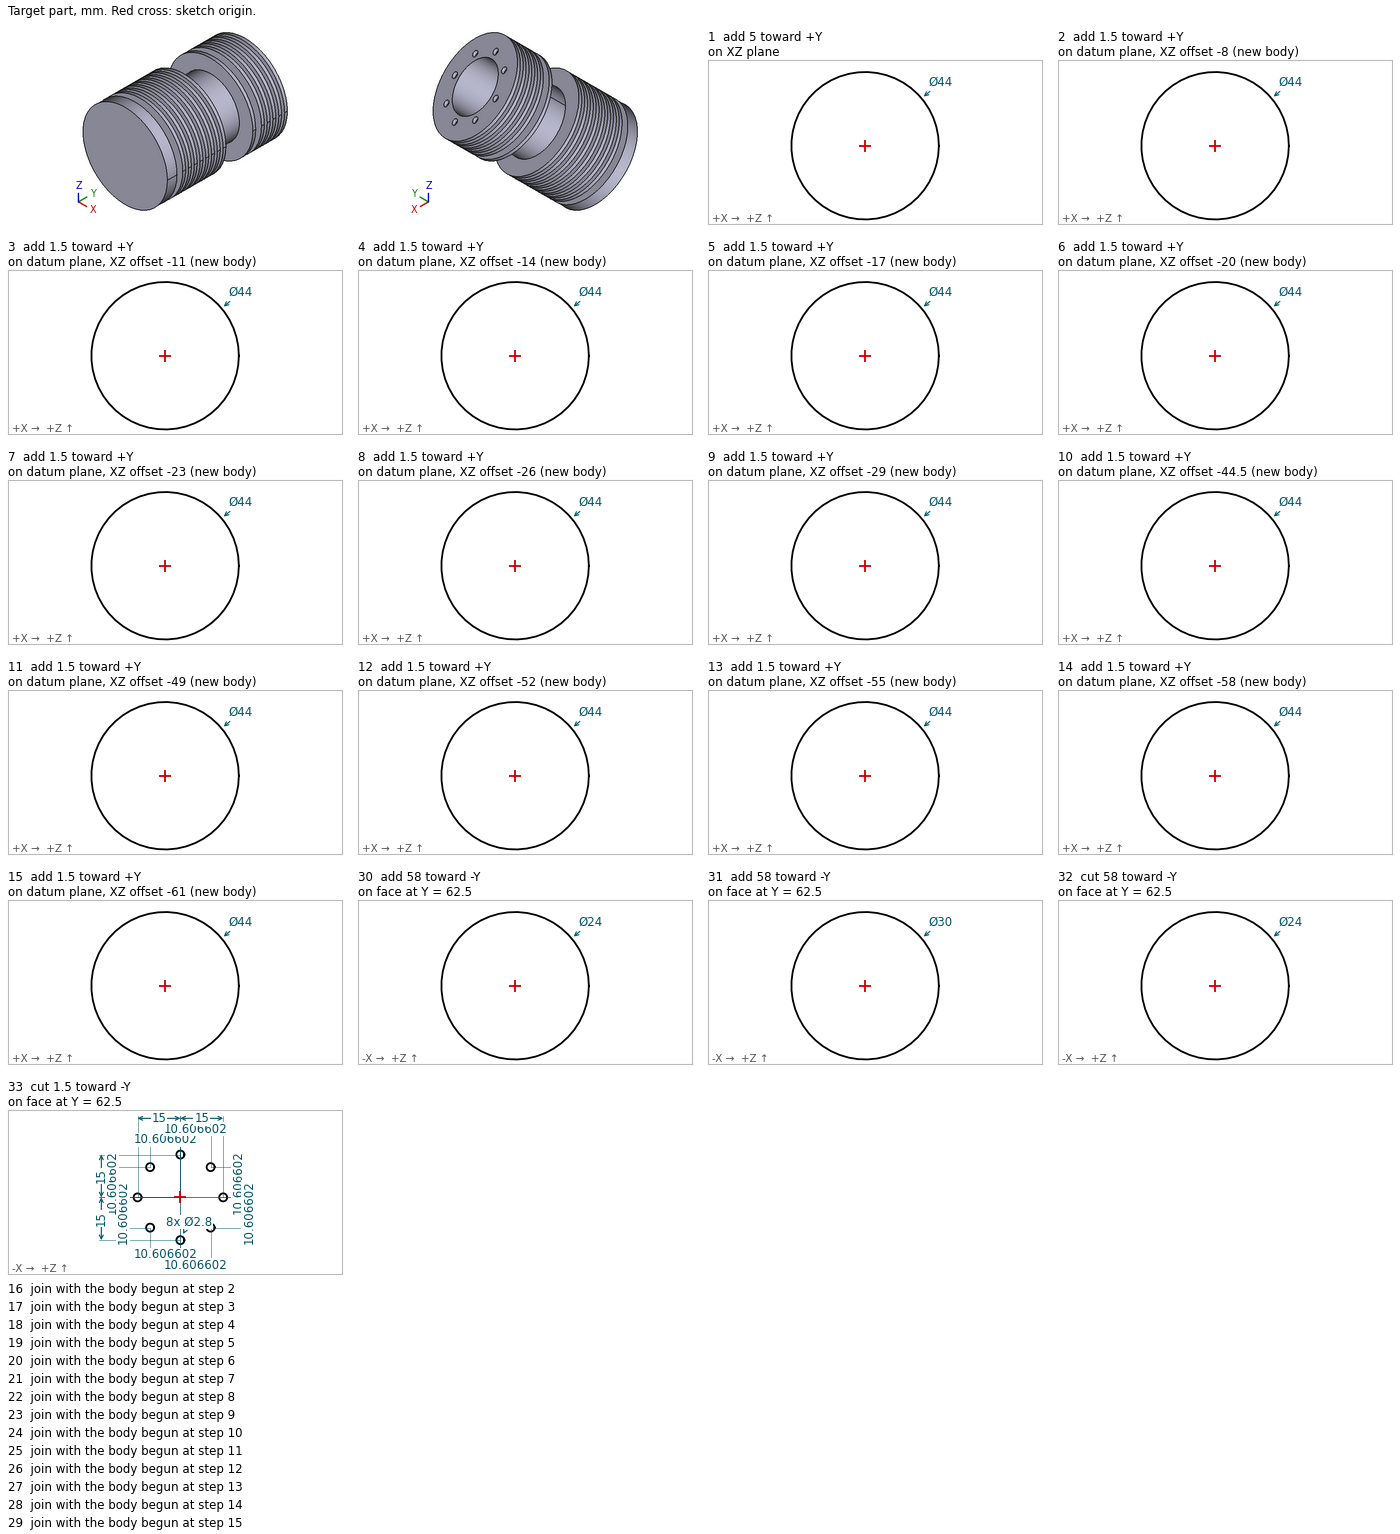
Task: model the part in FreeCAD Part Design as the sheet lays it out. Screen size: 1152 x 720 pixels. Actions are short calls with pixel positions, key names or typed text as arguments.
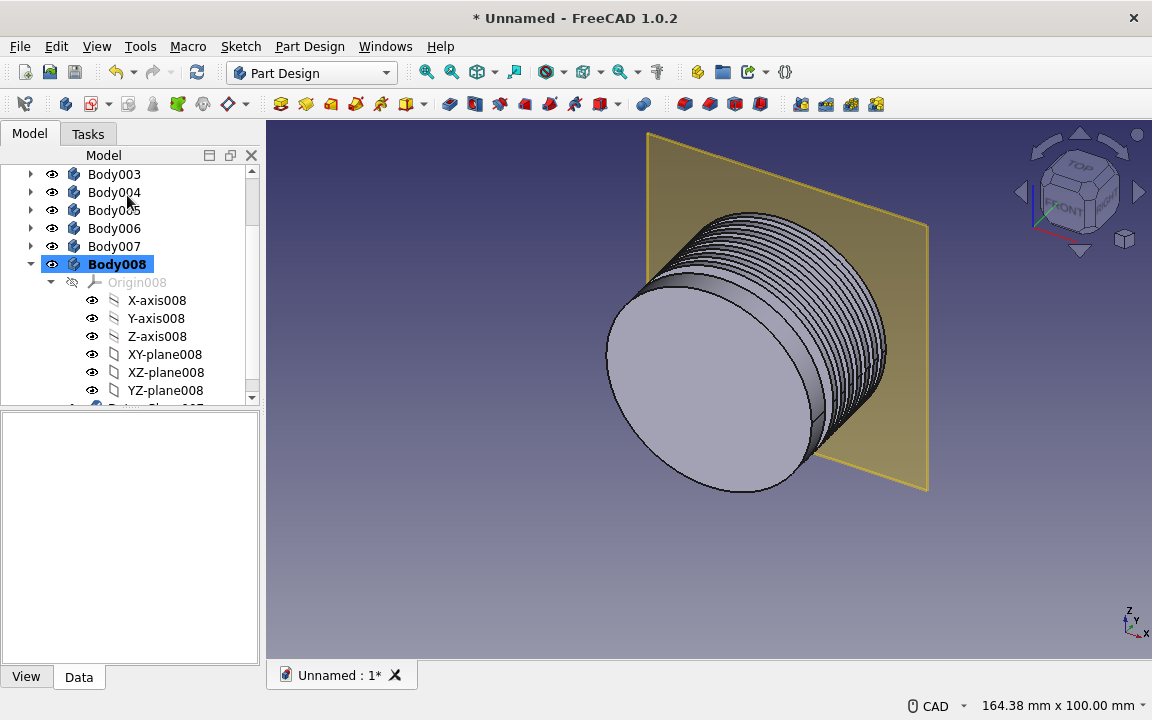
scroll(121, 278, down, 3)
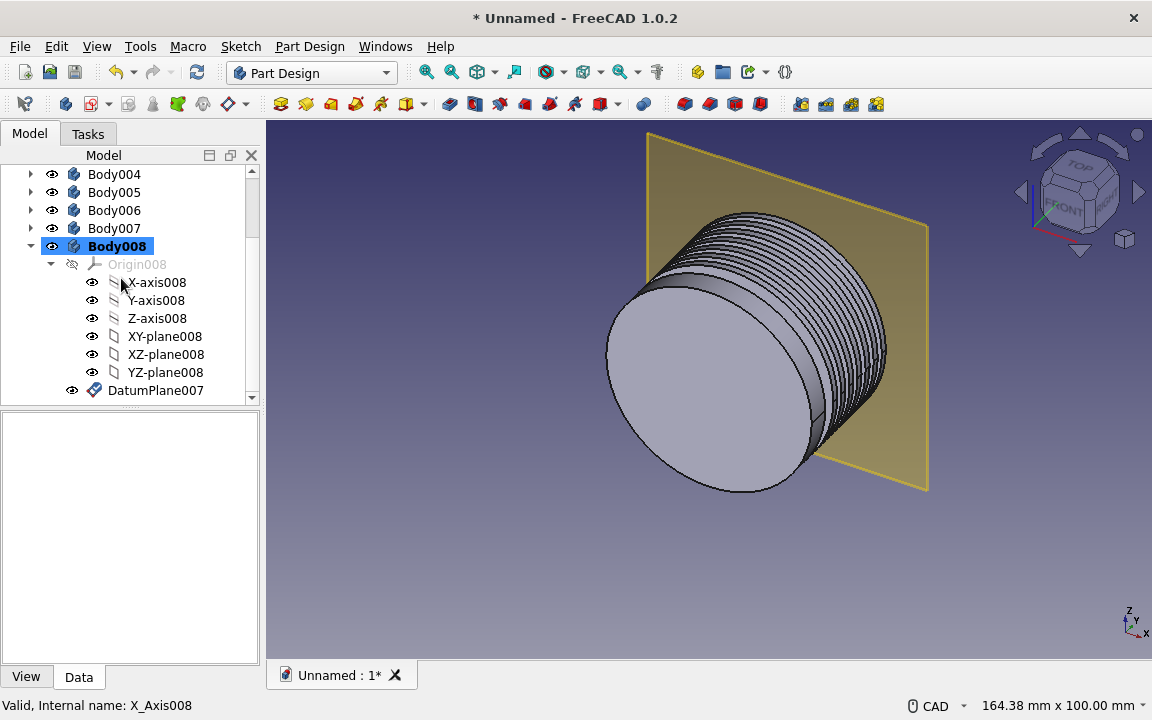
click(117, 390)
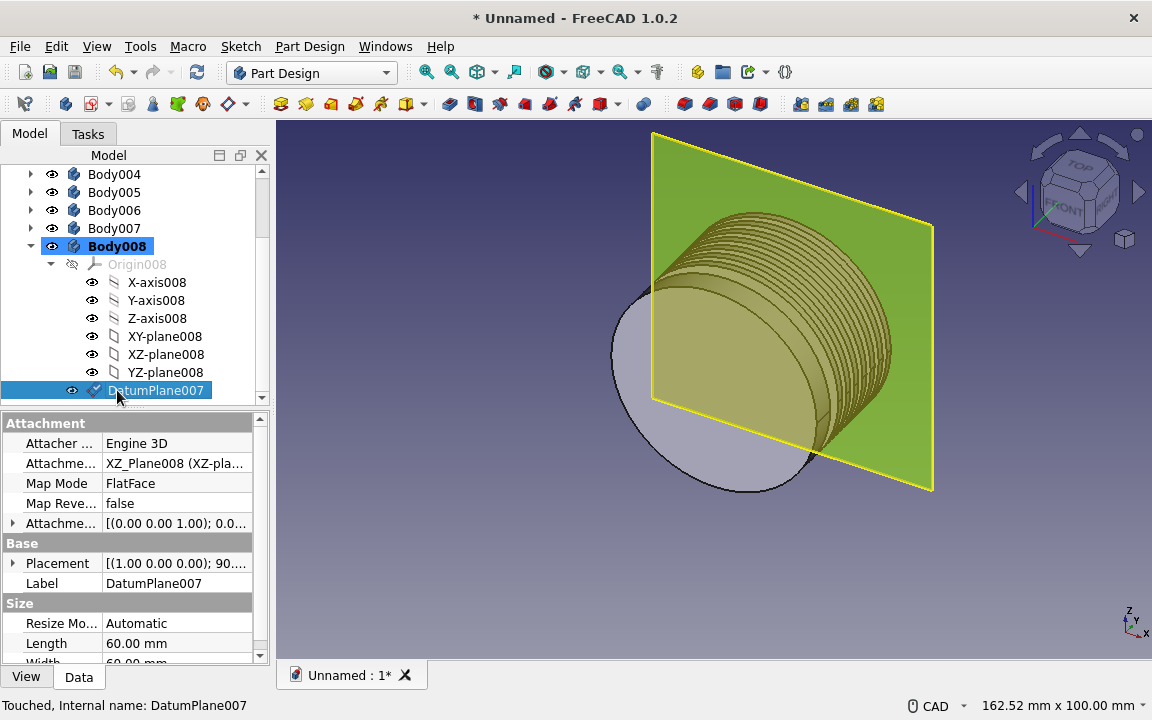
click(90, 104)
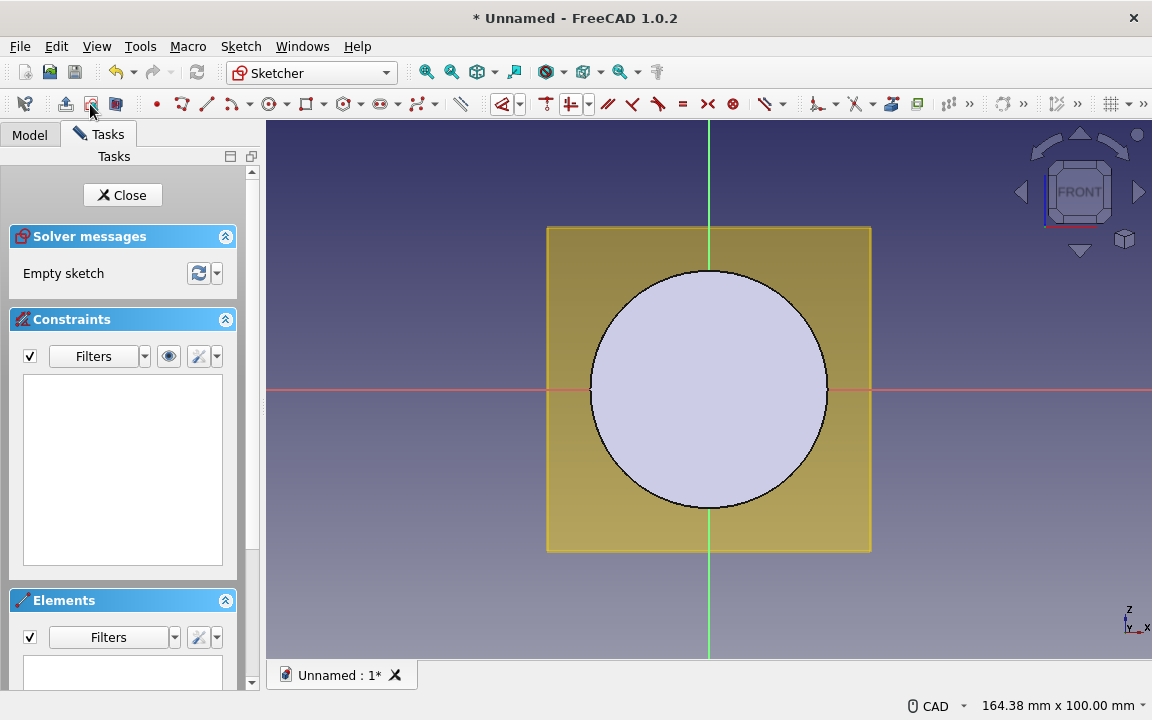
scroll(848, 390, up, 2)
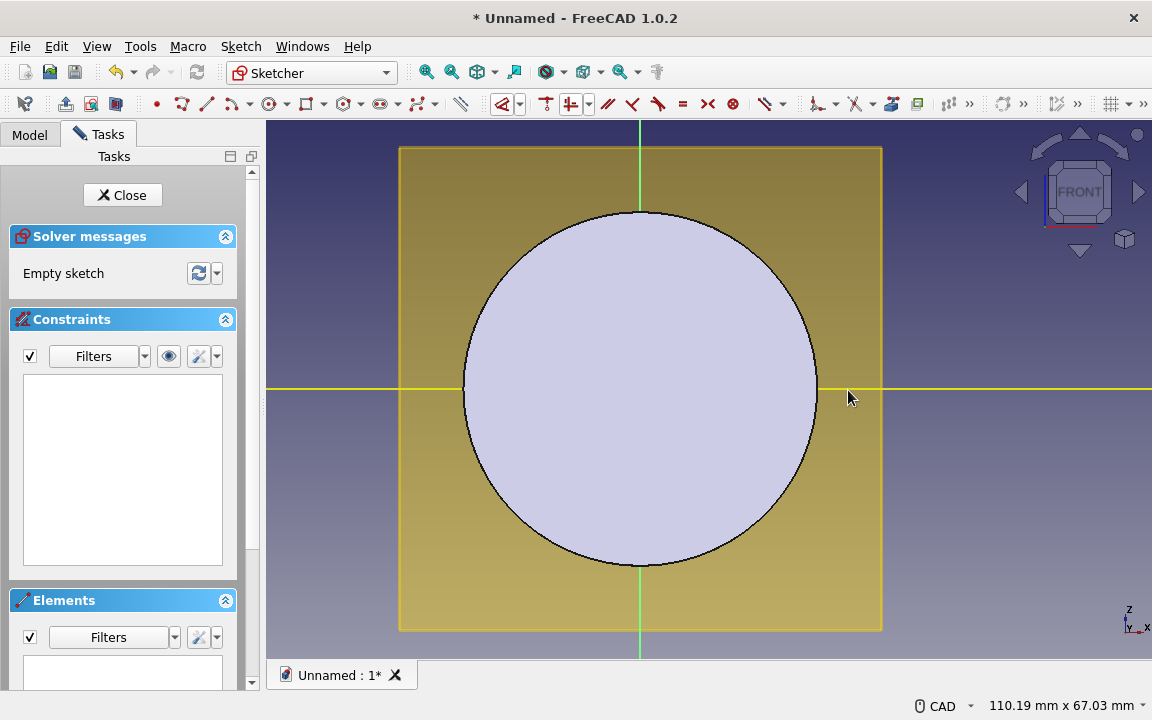
click(268, 104)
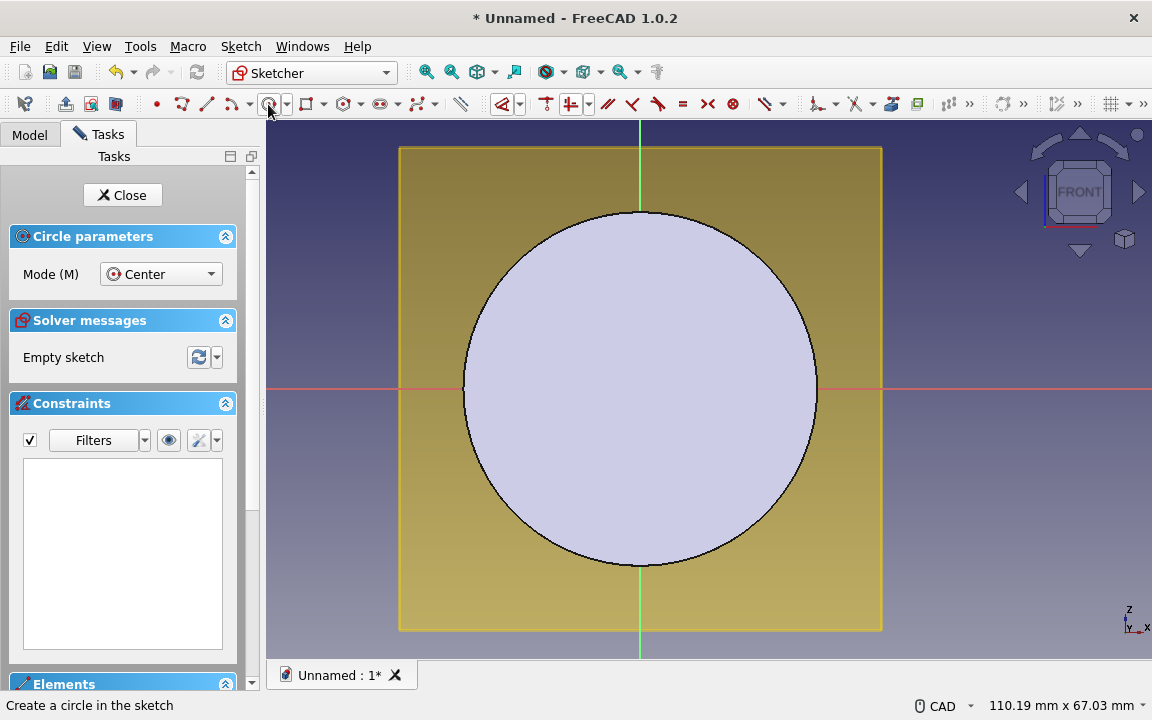
click(640, 389)
click(765, 264)
key(Escape)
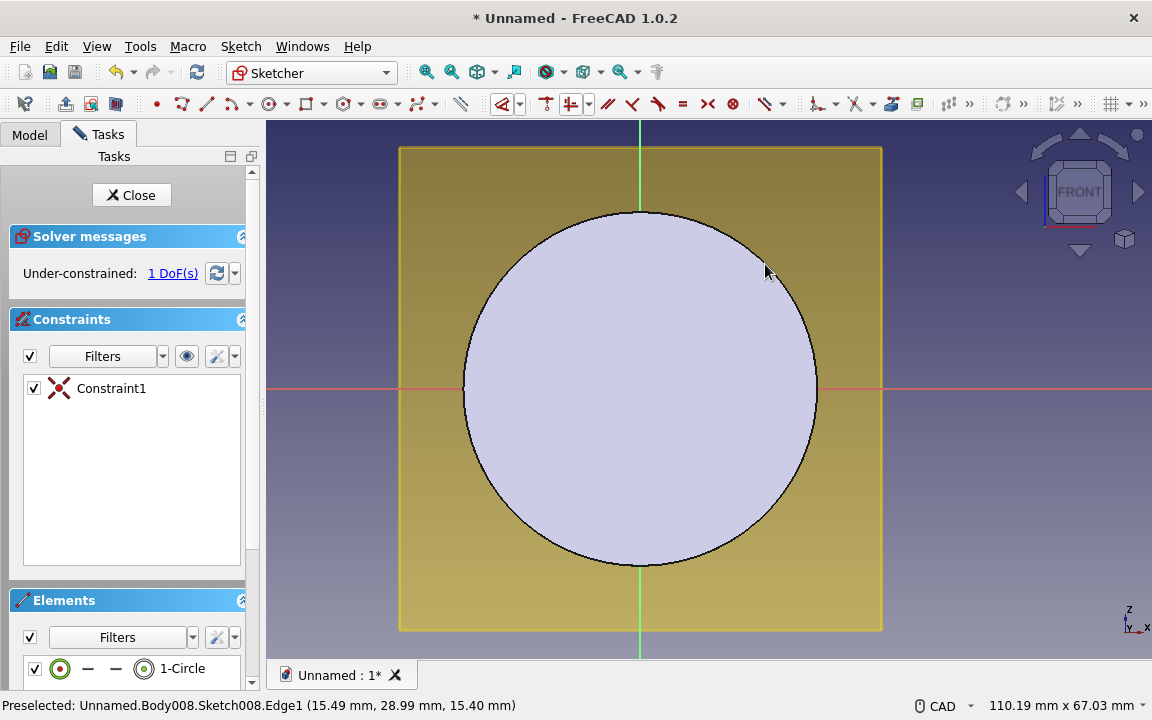
click(764, 264)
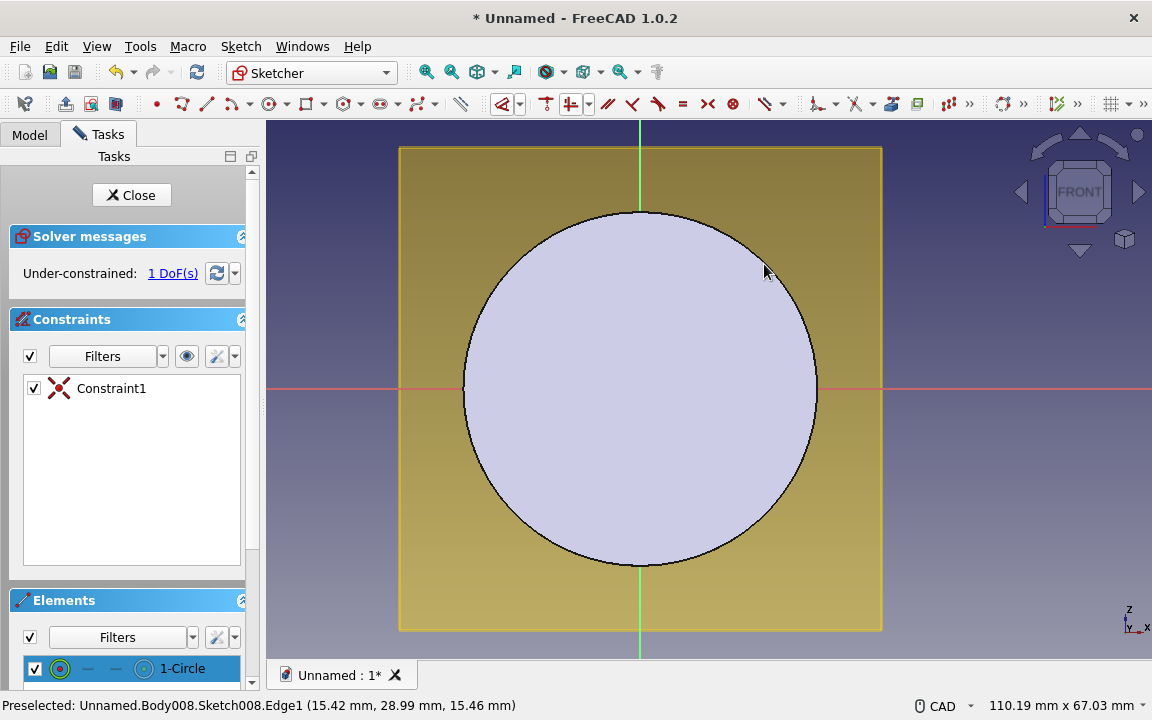
key(k)
key(o)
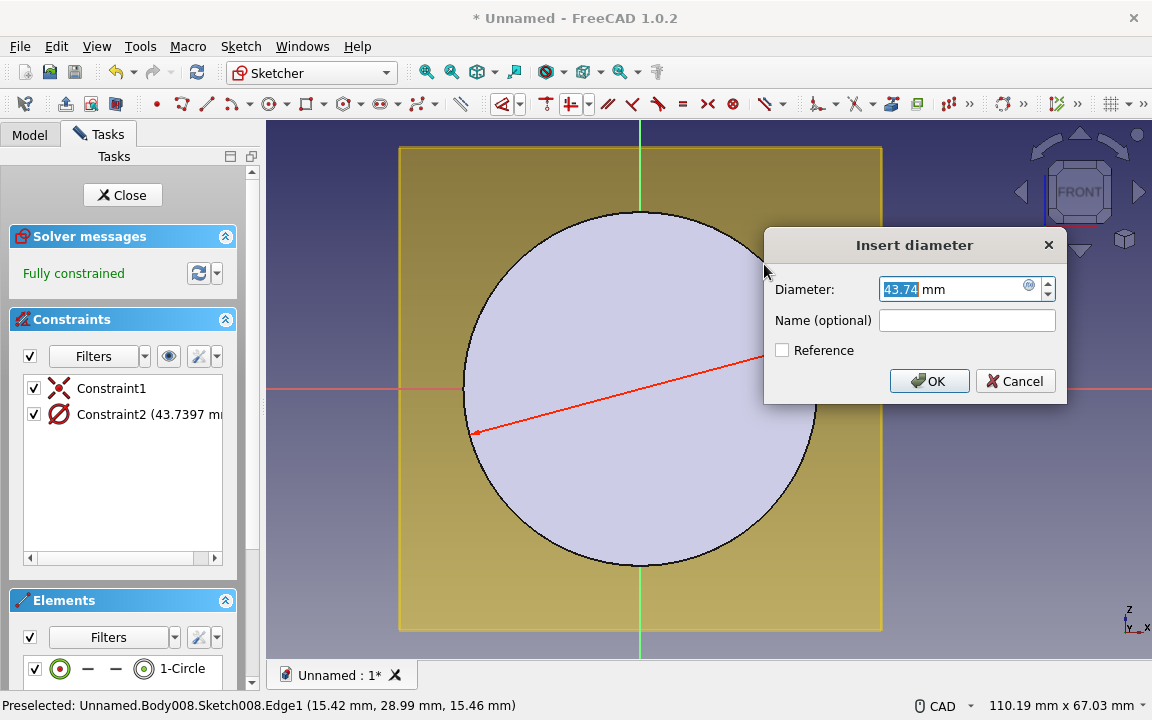
text(44)
key(Return)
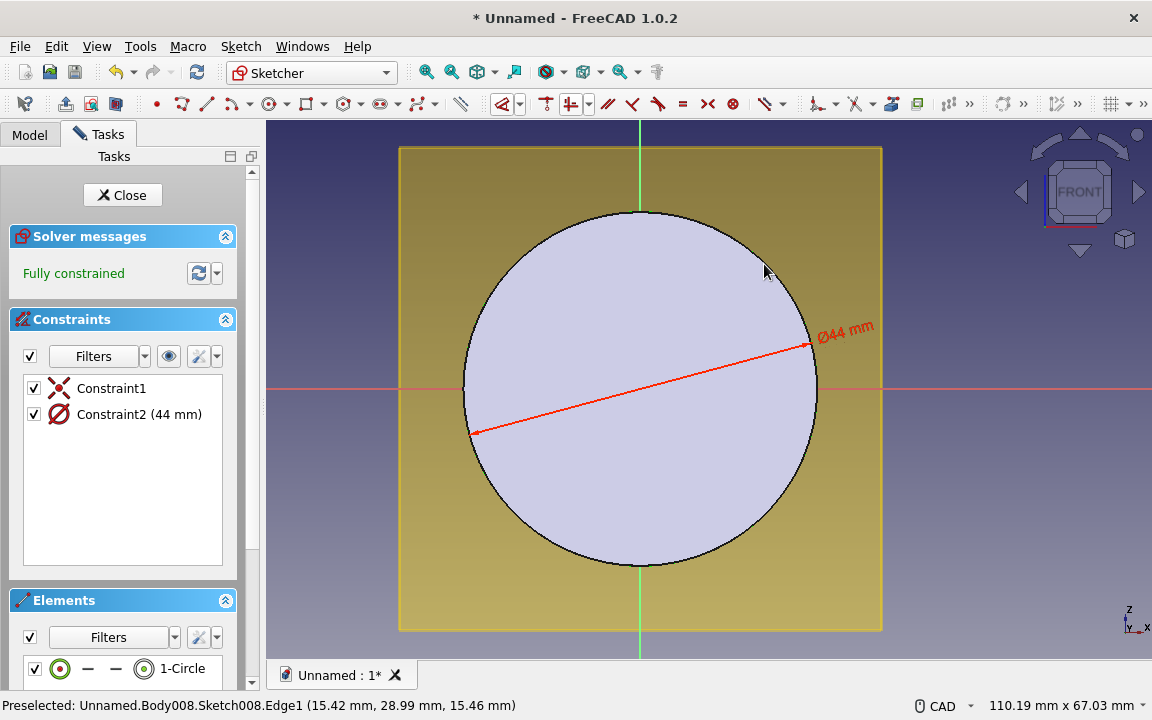
click(123, 195)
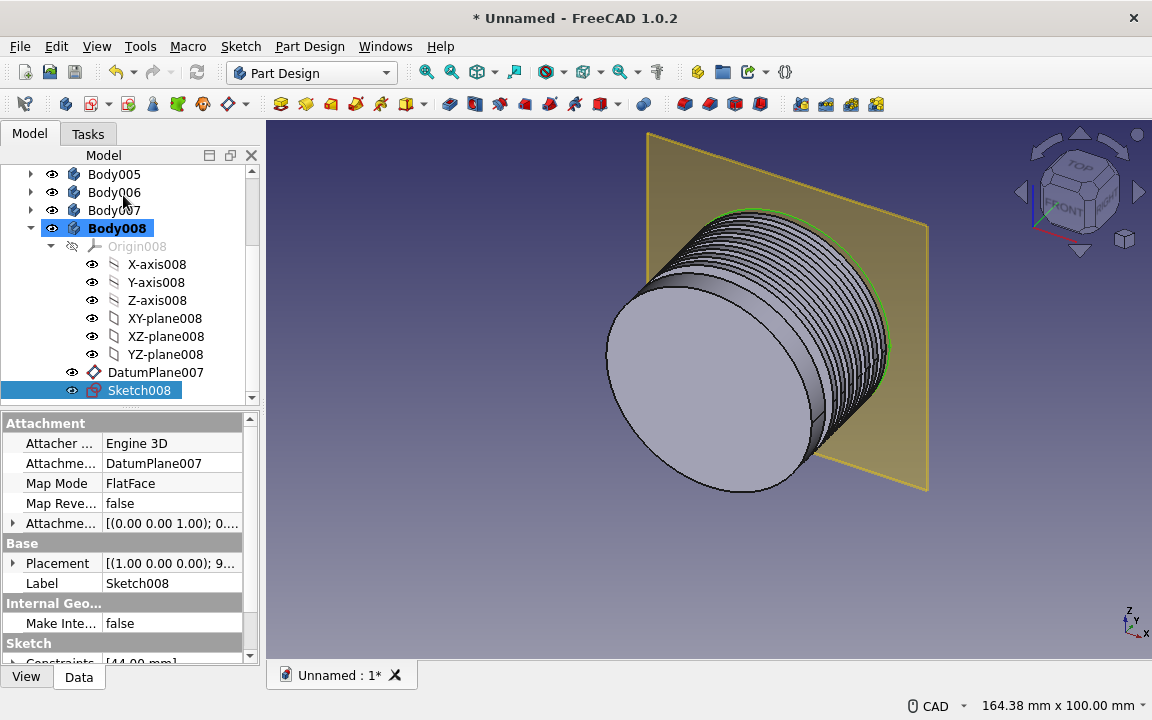
click(281, 104)